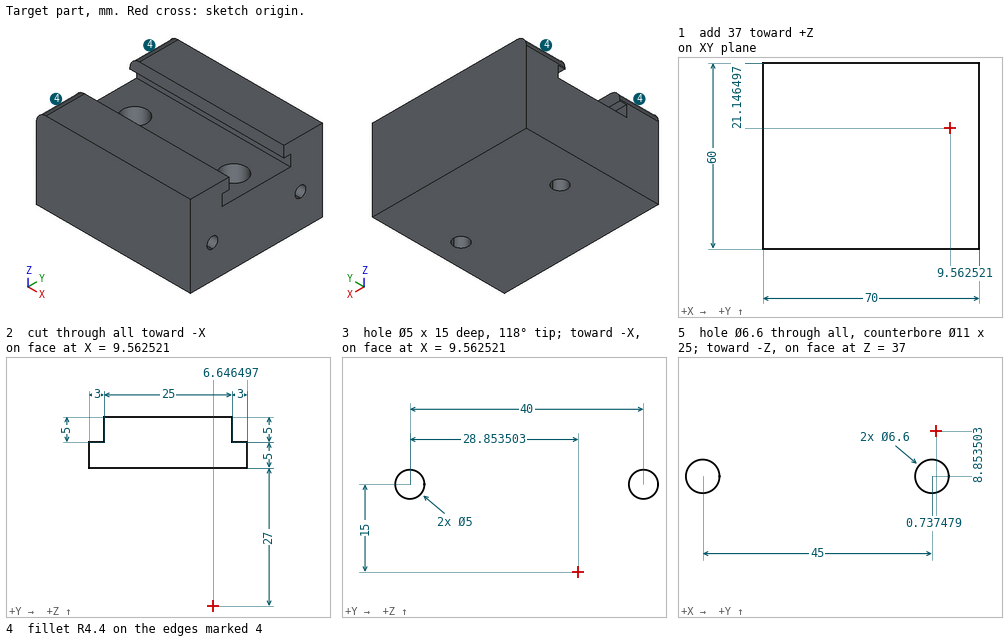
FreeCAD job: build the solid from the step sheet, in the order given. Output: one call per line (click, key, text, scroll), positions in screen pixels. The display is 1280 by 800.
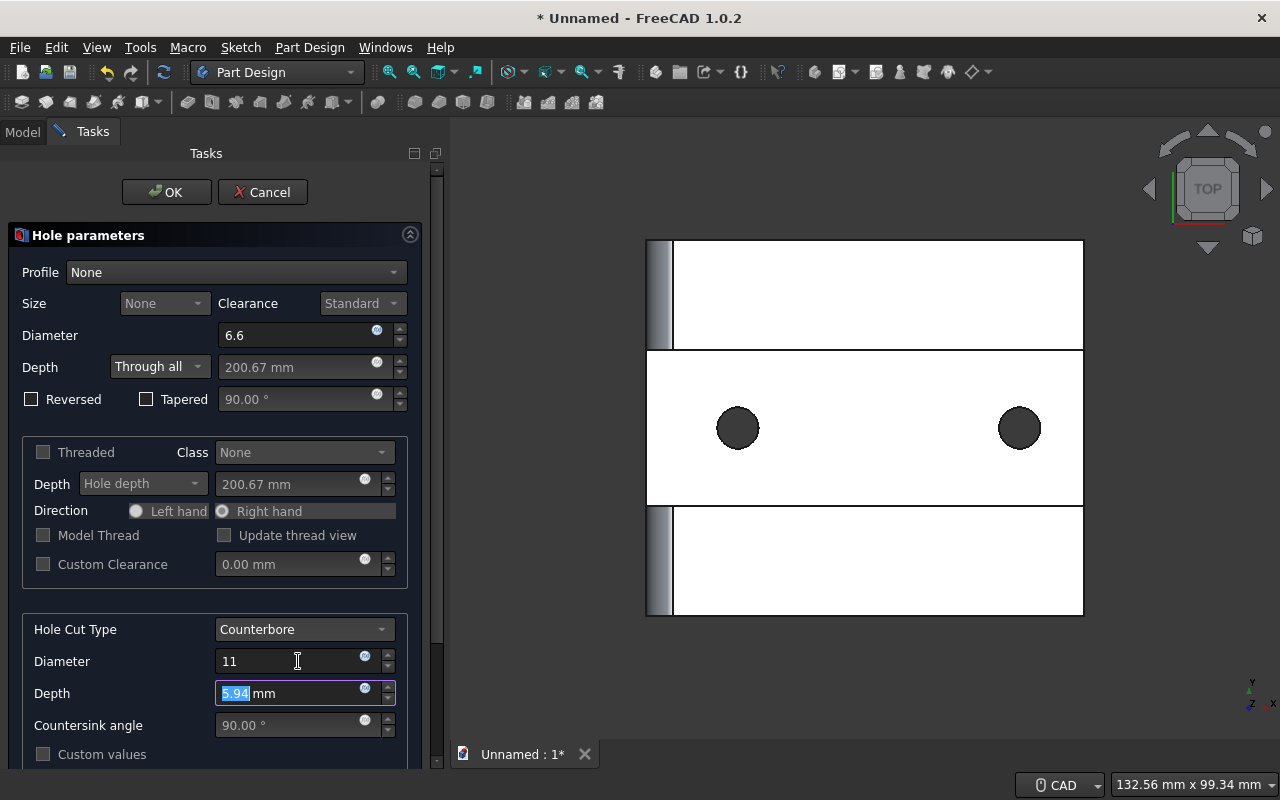
text(25)
key(Tab)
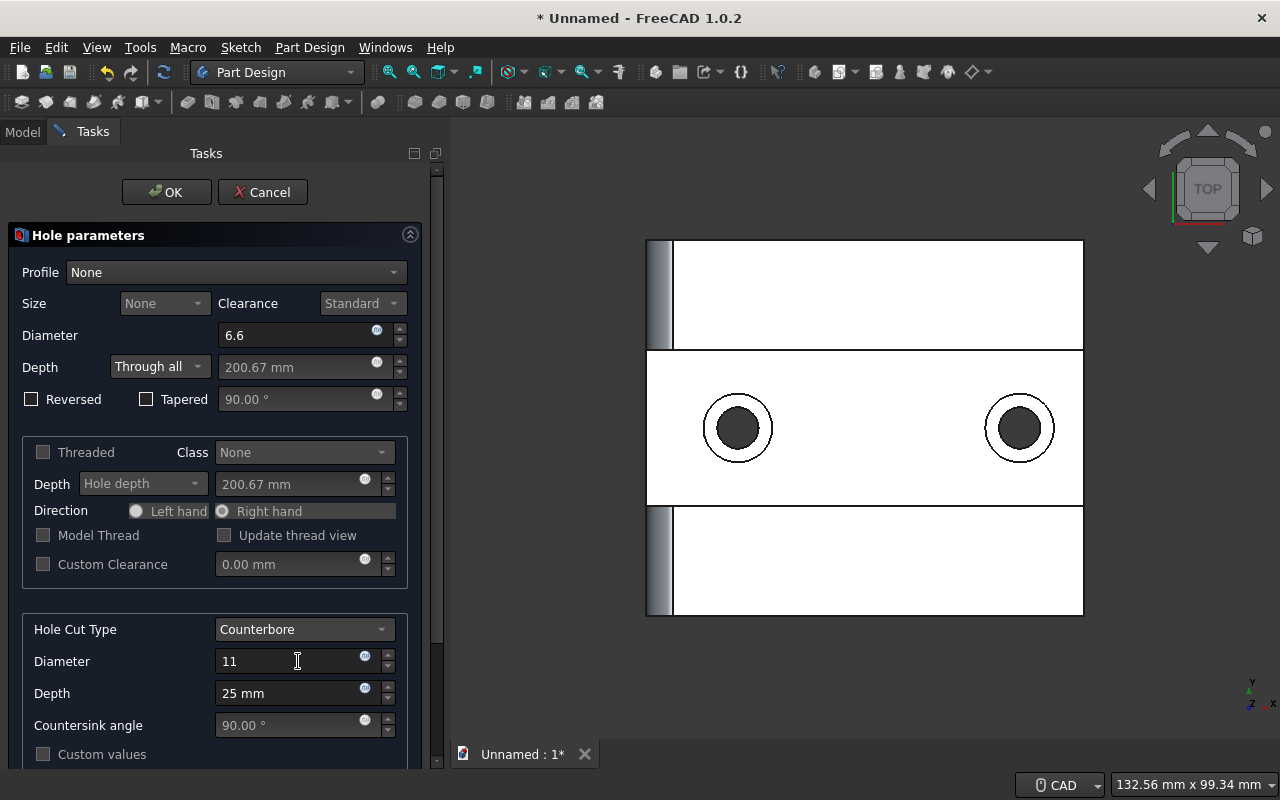
click(167, 192)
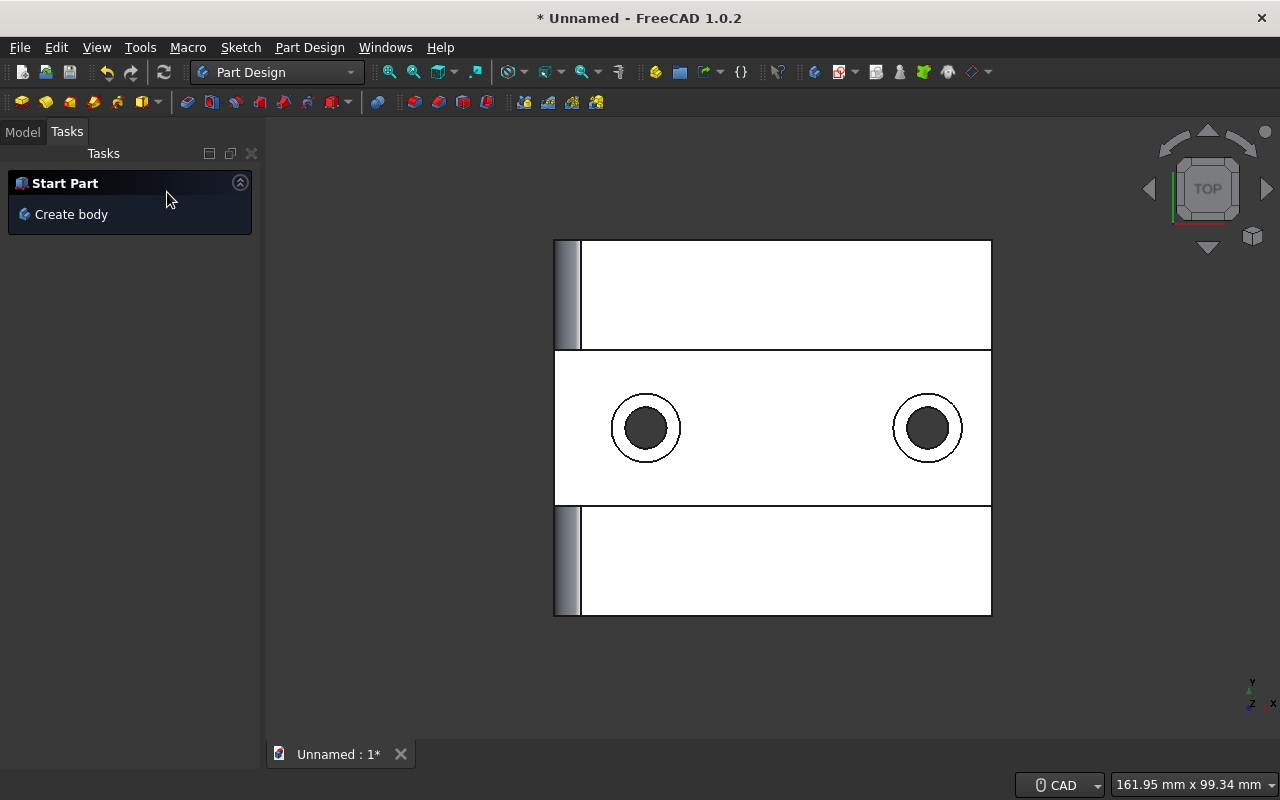
key(0)